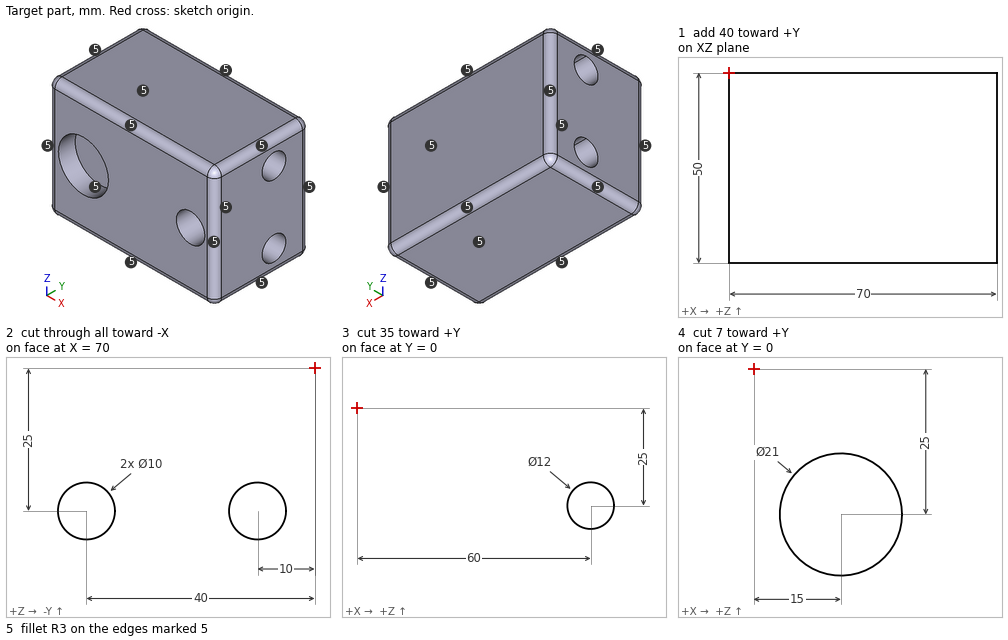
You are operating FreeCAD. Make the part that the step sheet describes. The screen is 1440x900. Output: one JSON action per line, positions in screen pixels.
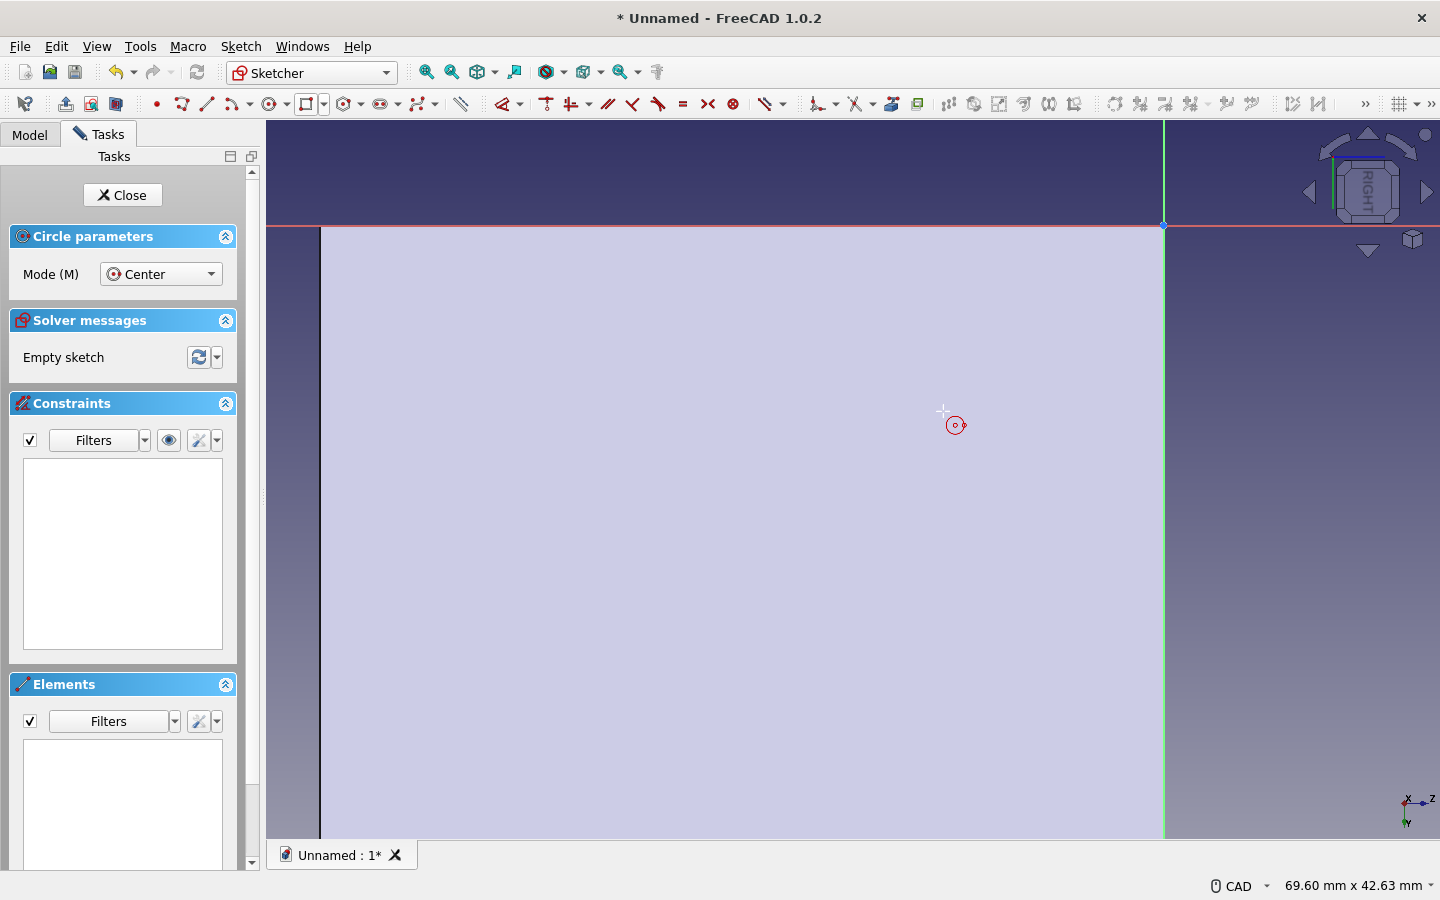
{"action": "left_click", "coordinate": [489, 647]}
{"action": "left_click", "coordinate": [549, 588]}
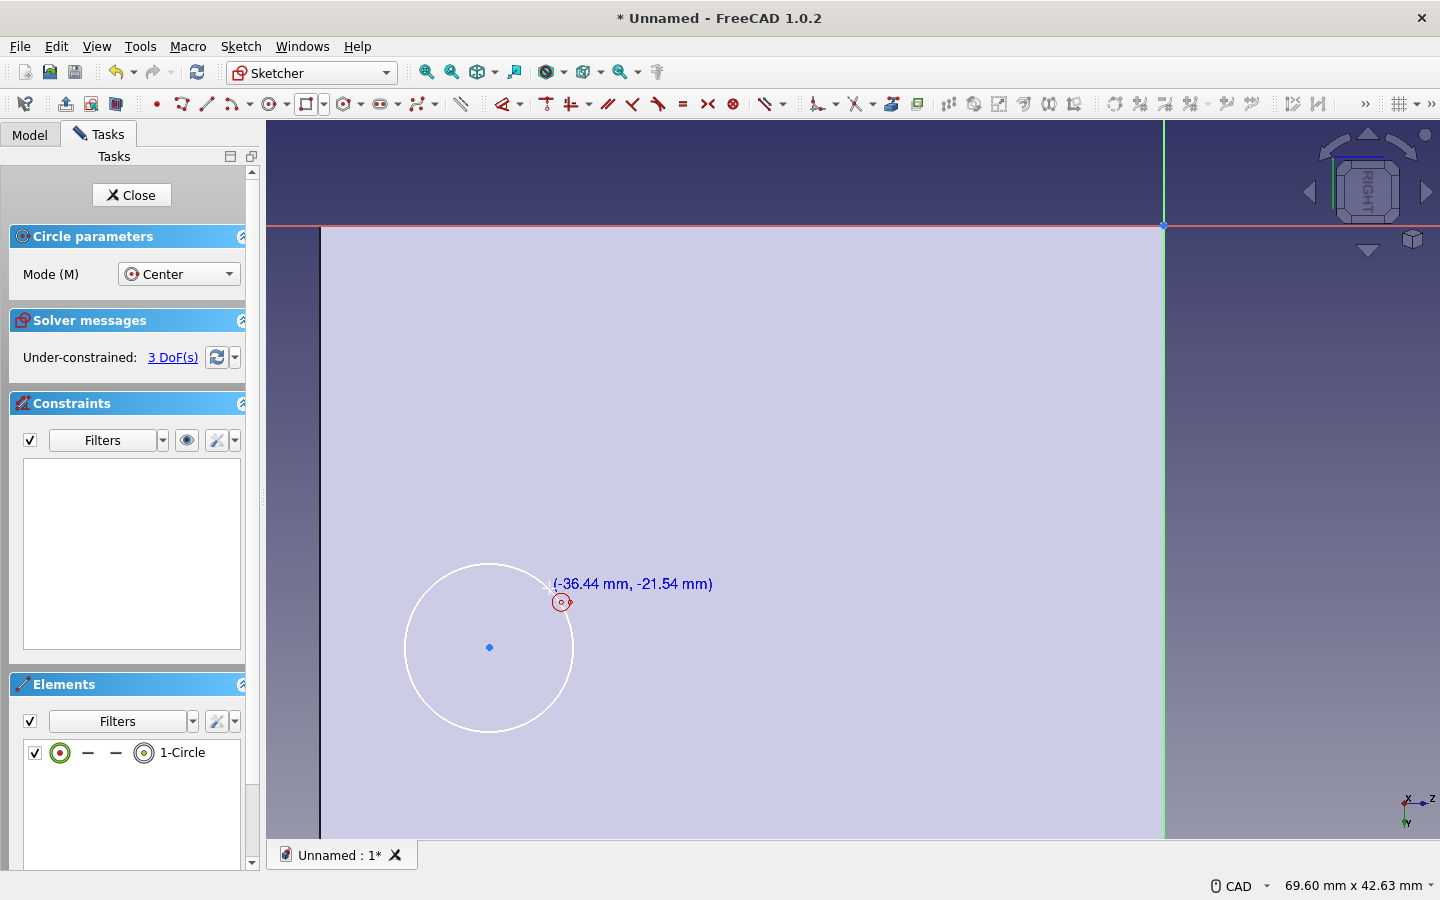
{"action": "left_click", "coordinate": [995, 647]}
{"action": "left_click", "coordinate": [1055, 588]}
{"action": "key", "text": "Escape"}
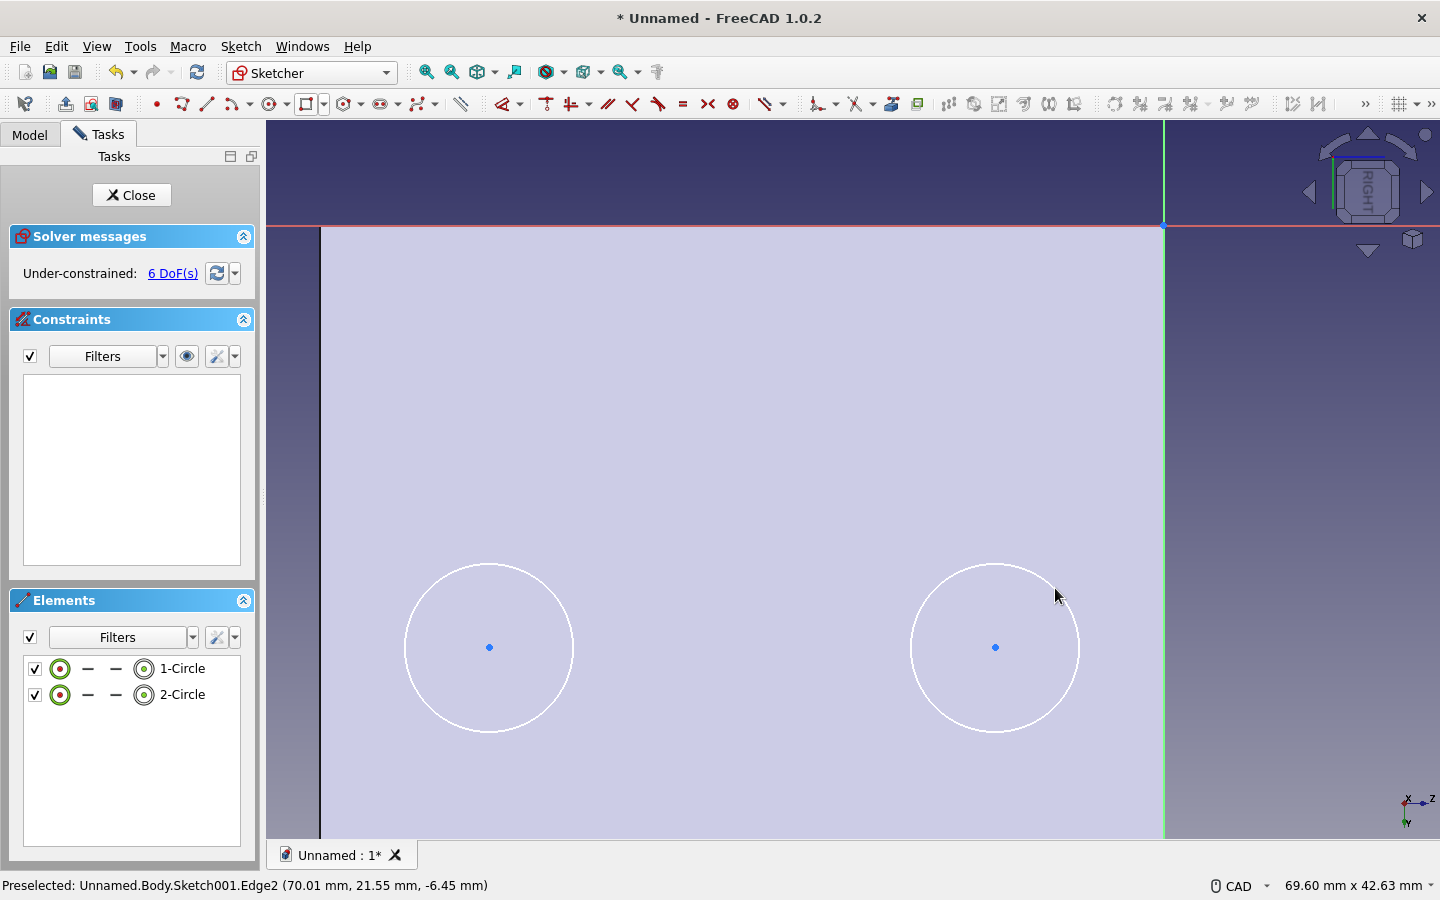
{"action": "left_click", "coordinate": [548, 588]}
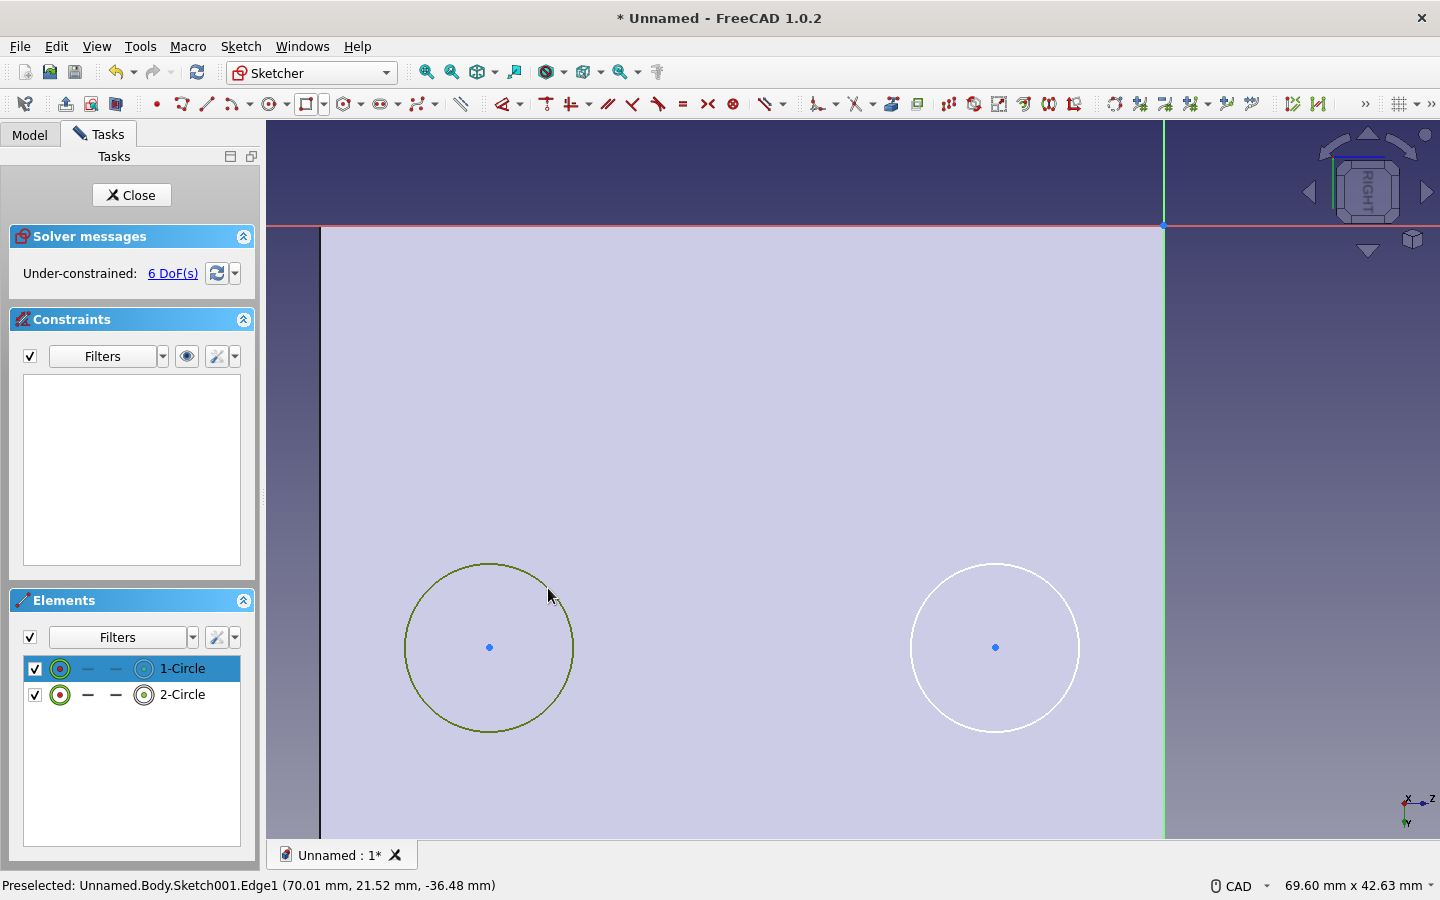
{"action": "left_click", "coordinate": [1054, 588]}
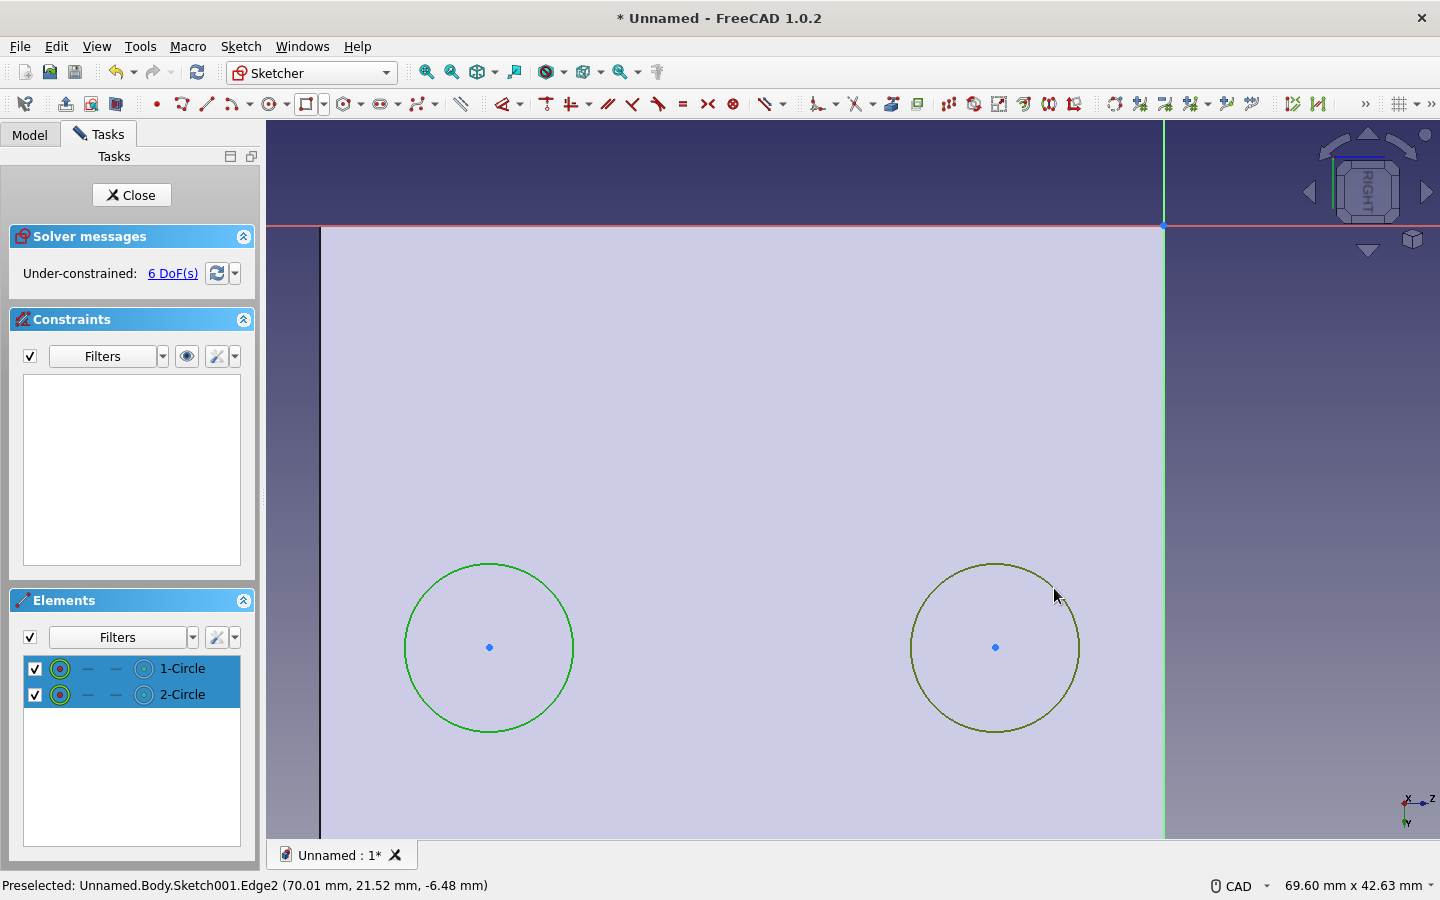
{"action": "left_click", "coordinate": [683, 104]}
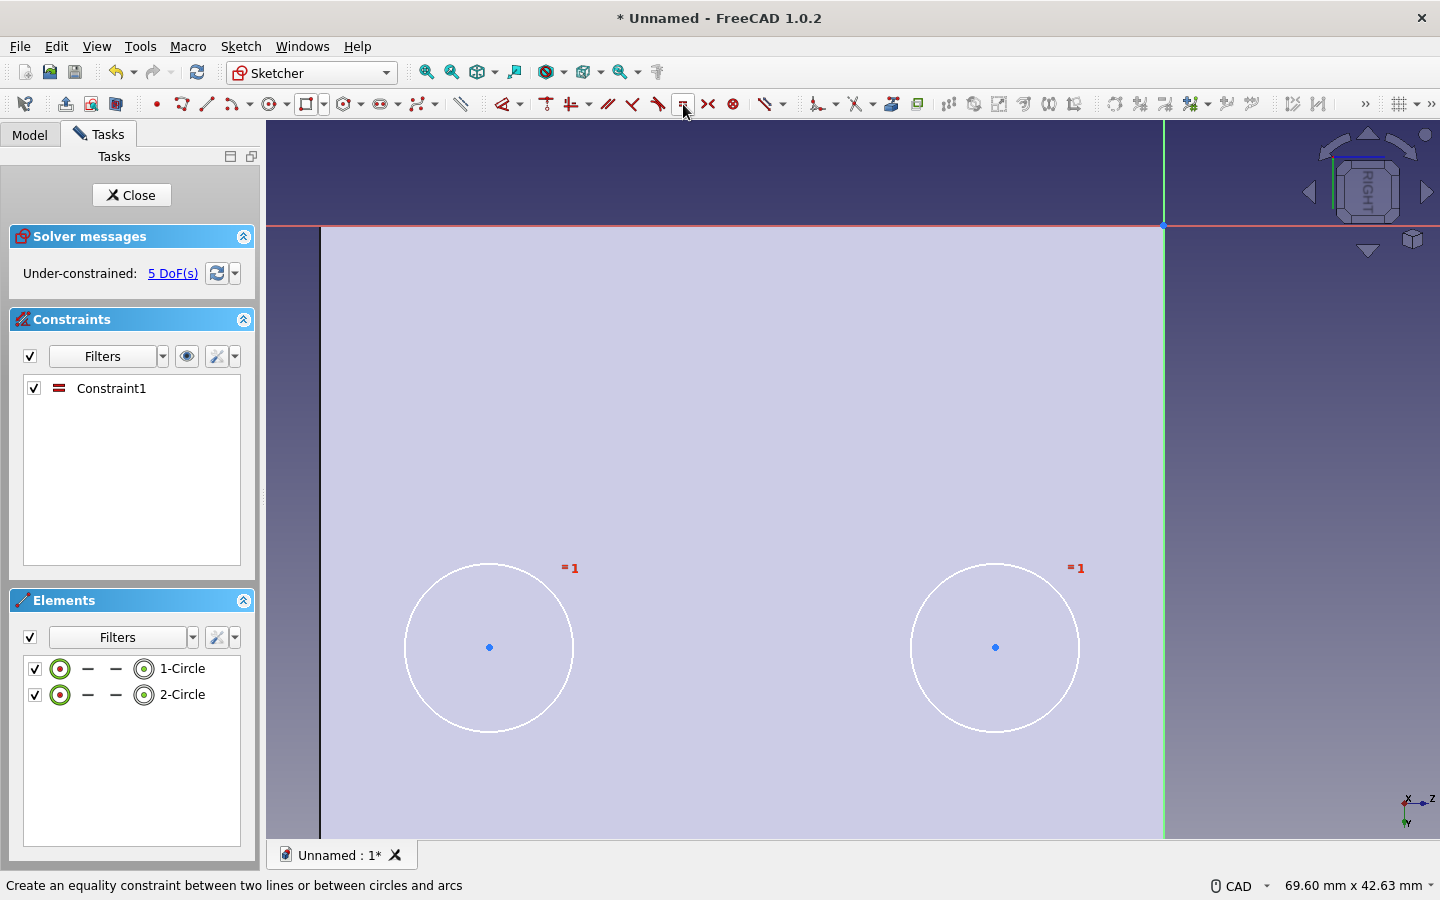
{"action": "left_click", "coordinate": [489, 648]}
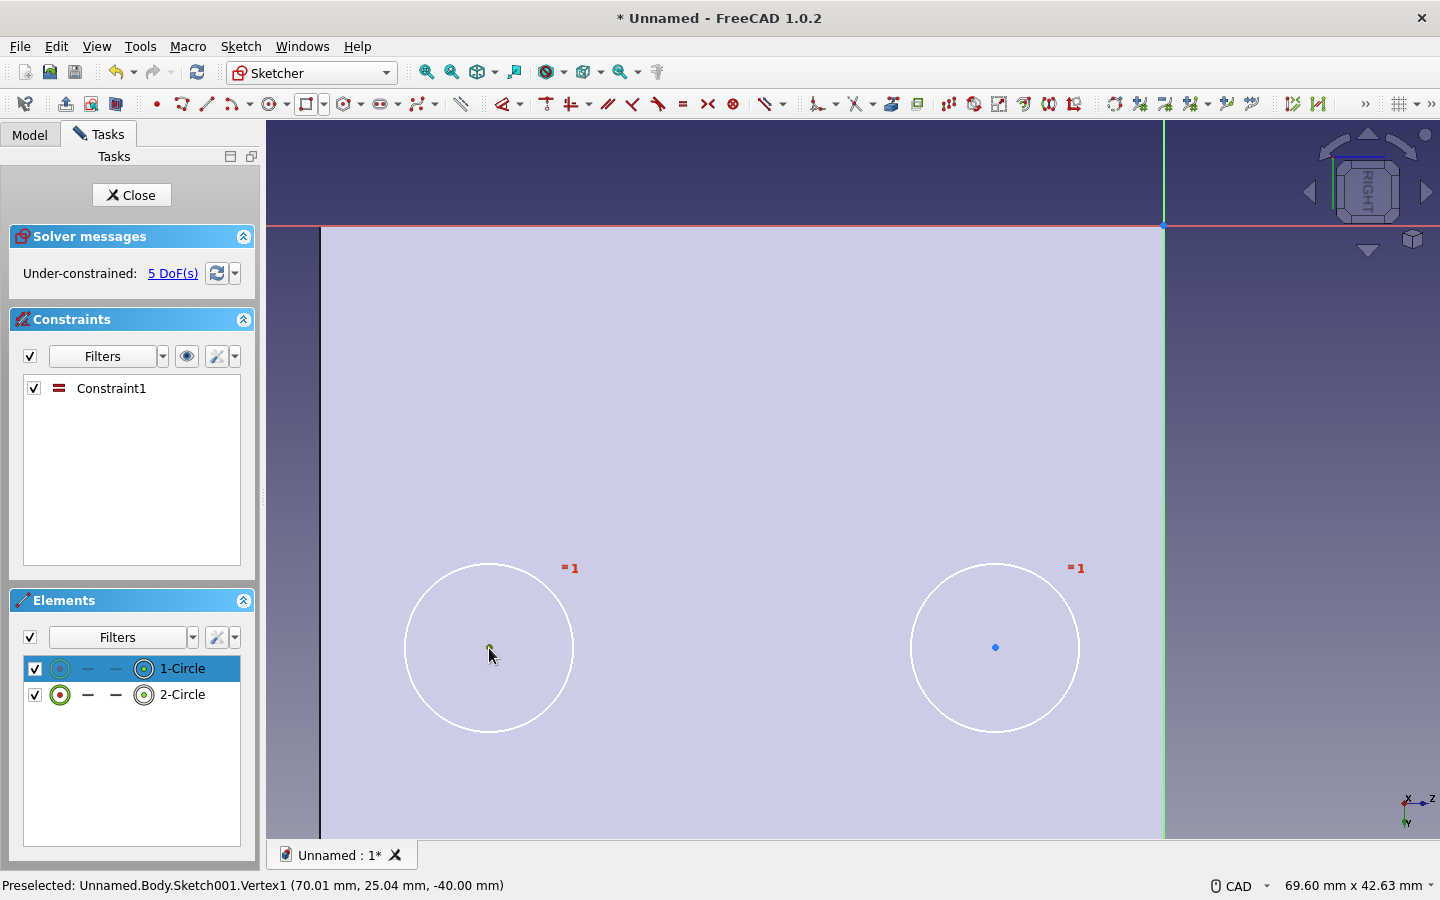
{"action": "left_click", "coordinate": [995, 648]}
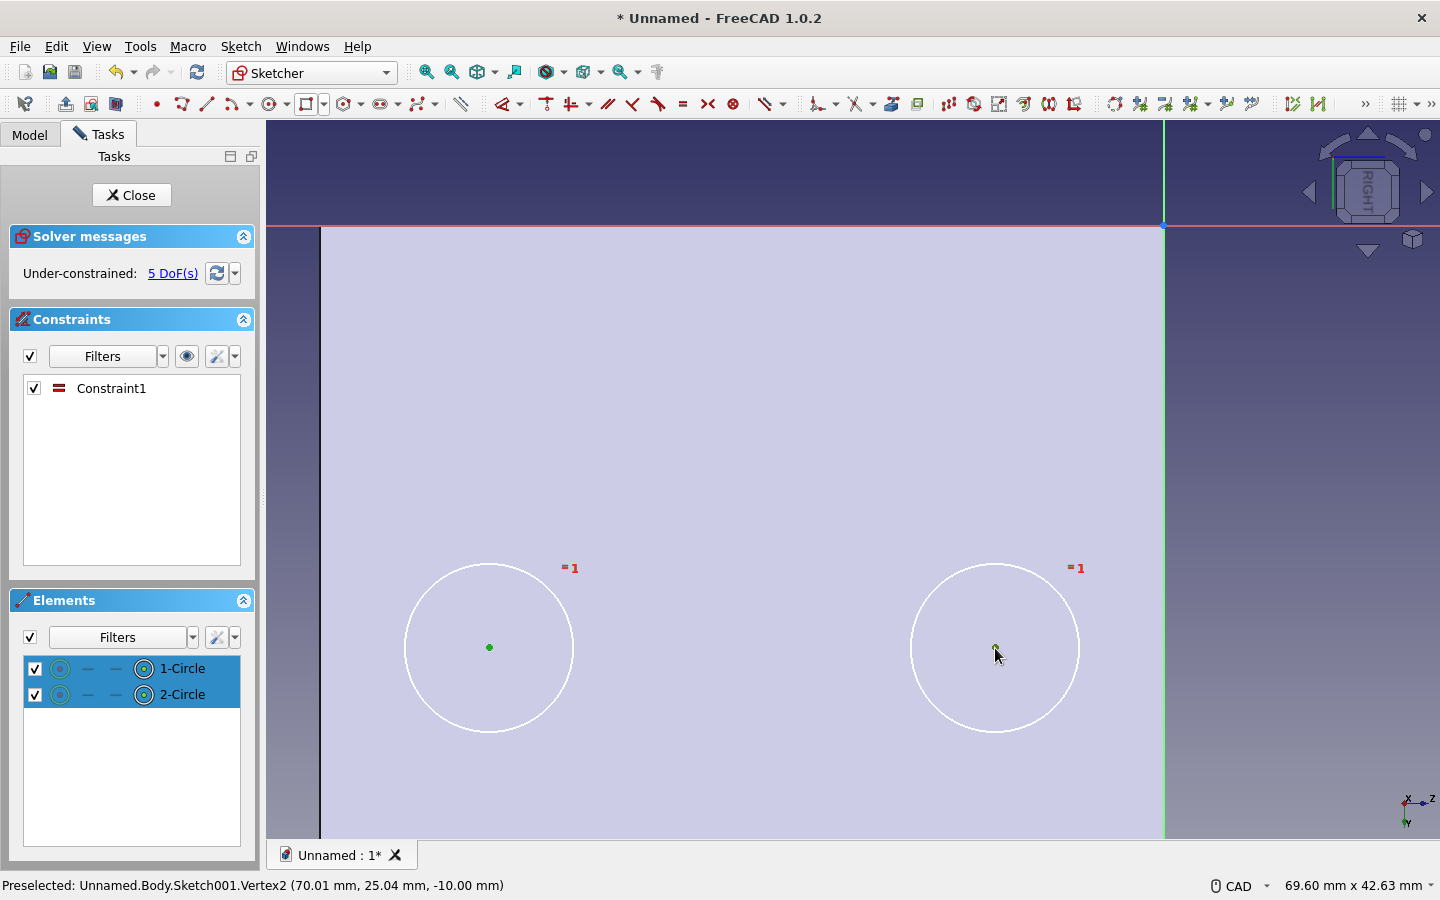
{"action": "key", "text": "h"}